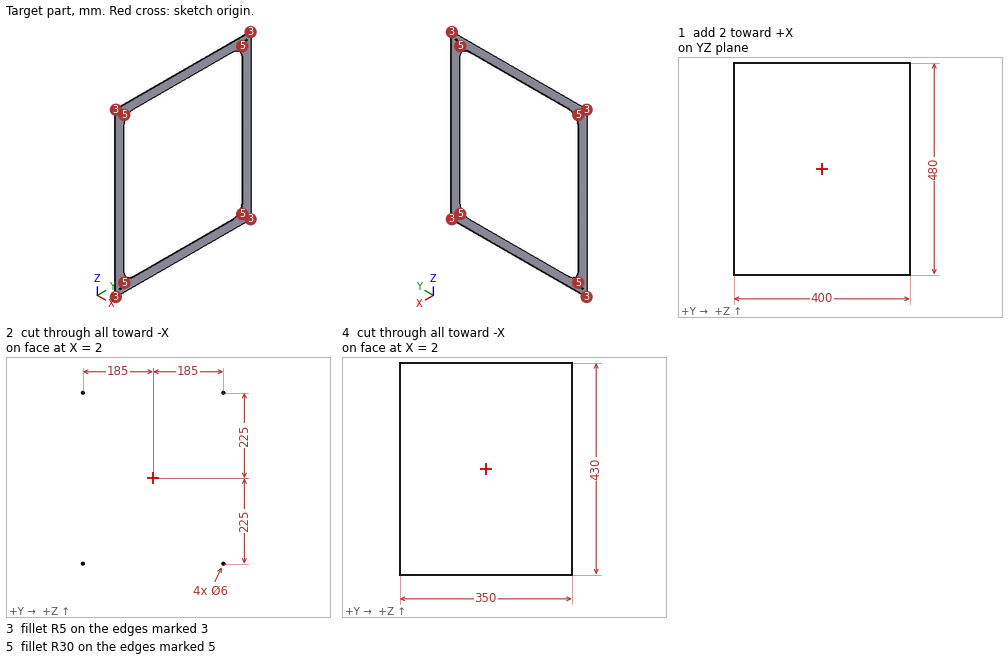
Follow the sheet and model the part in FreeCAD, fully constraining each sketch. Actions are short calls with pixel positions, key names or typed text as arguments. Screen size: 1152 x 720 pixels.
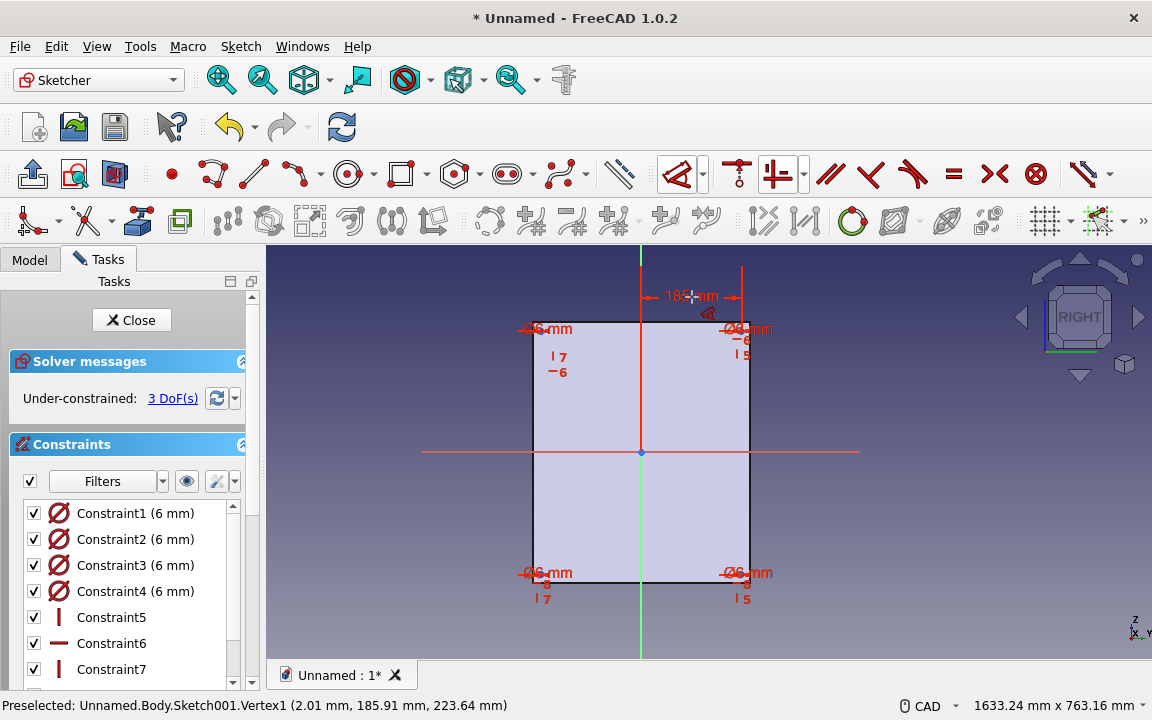
click(742, 331)
click(776, 392)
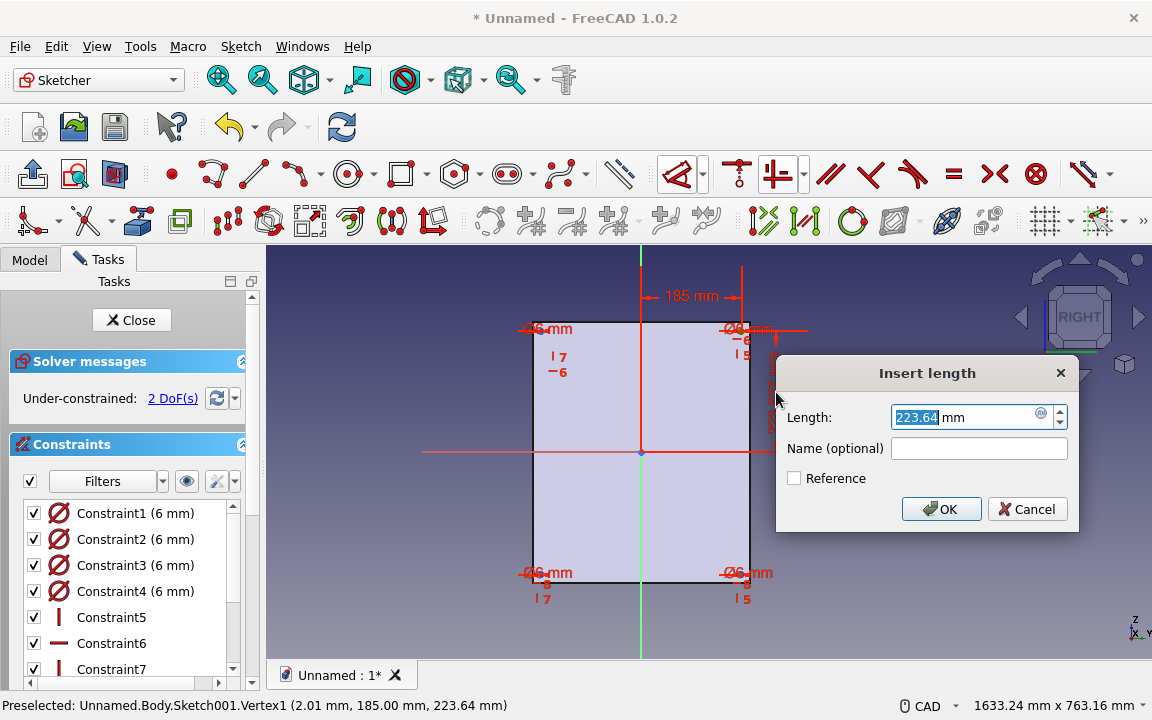
text(225)
key(Return)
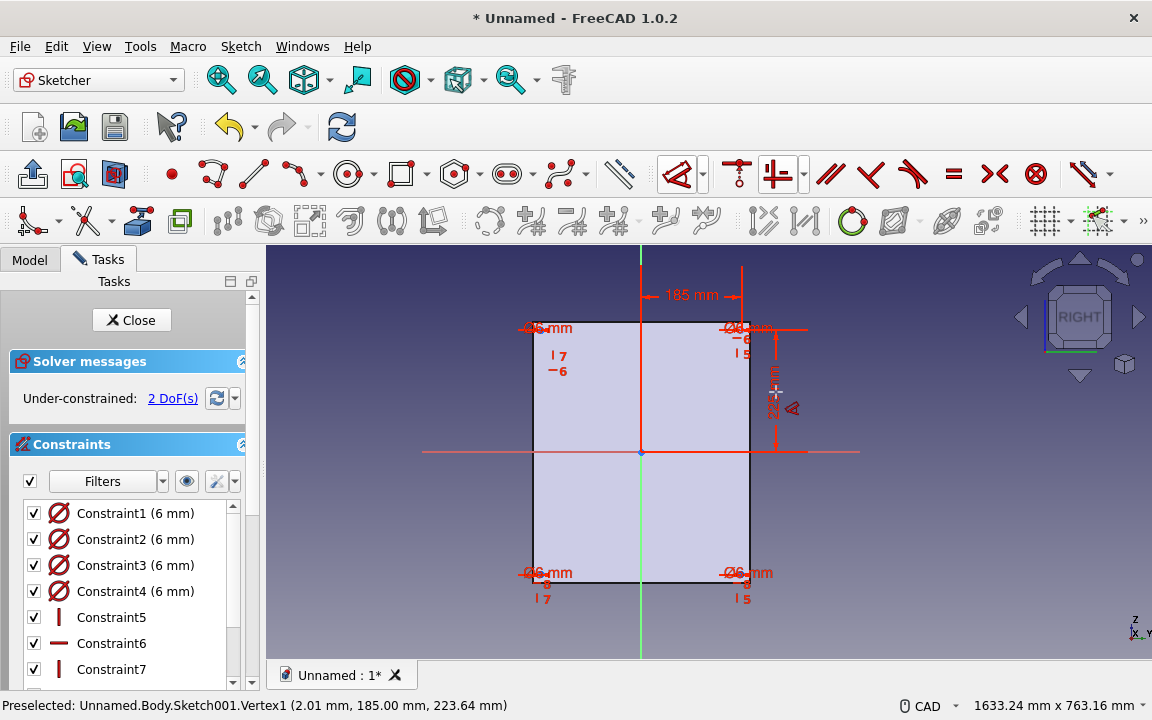
click(742, 575)
click(776, 514)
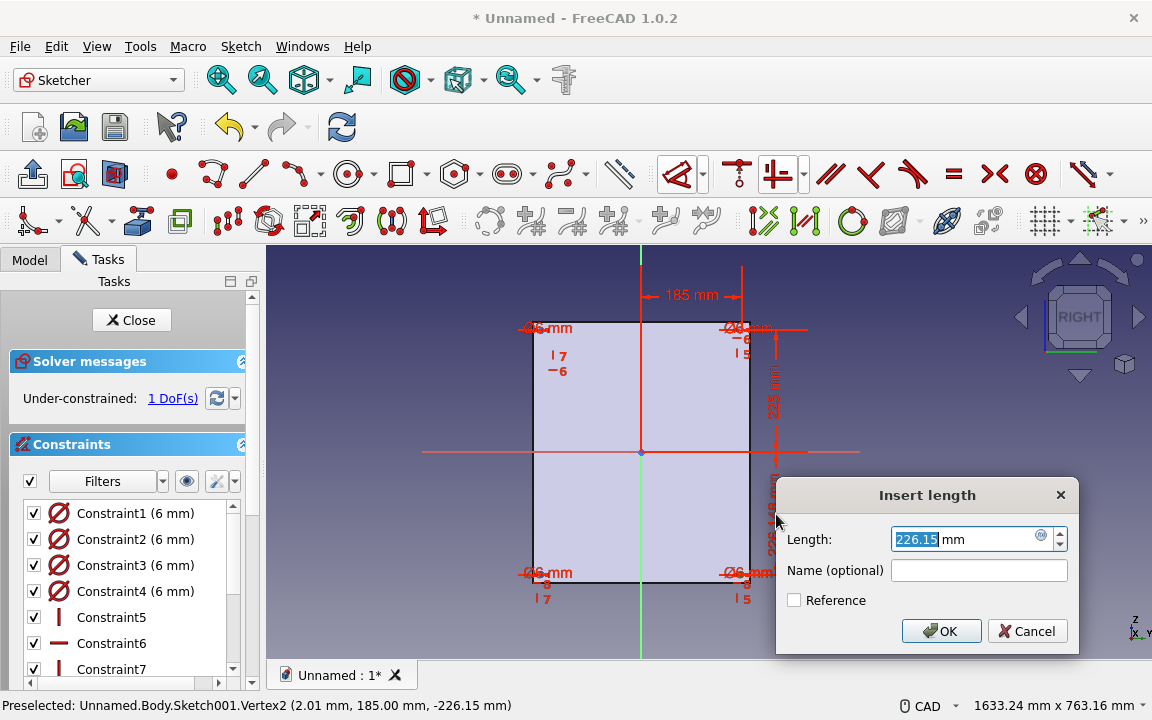
text(225)
key(Return)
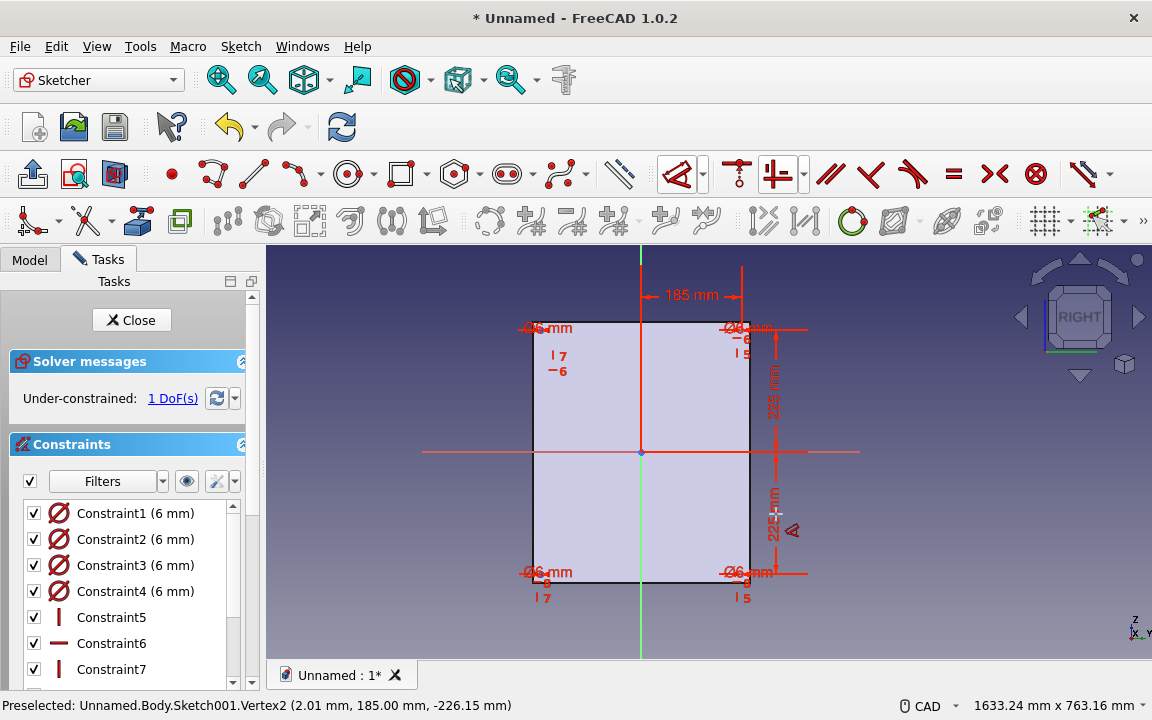
click(541, 330)
click(591, 296)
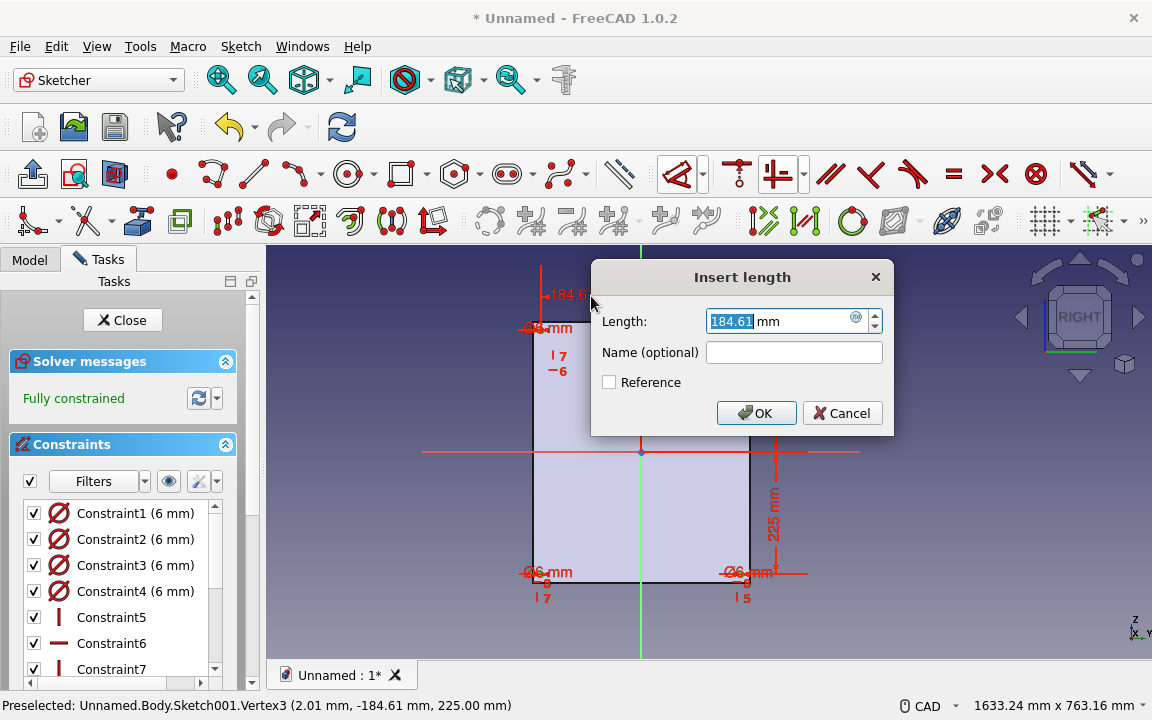
text(185)
key(Return)
key(Escape)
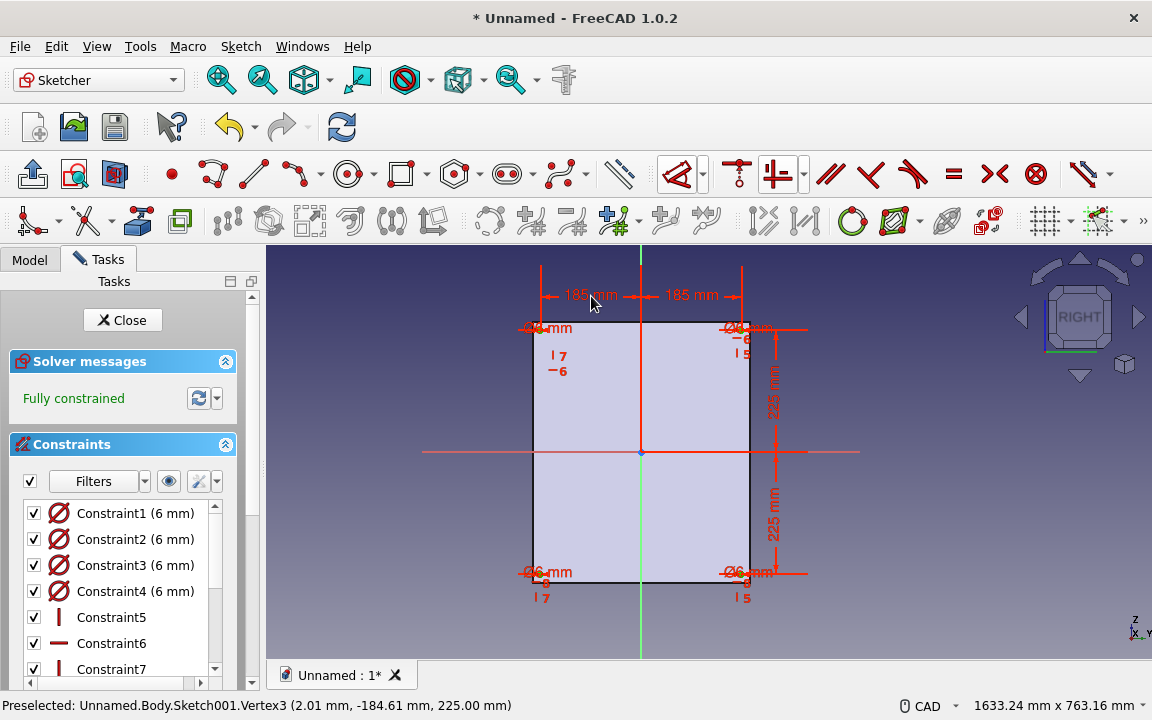
click(123, 320)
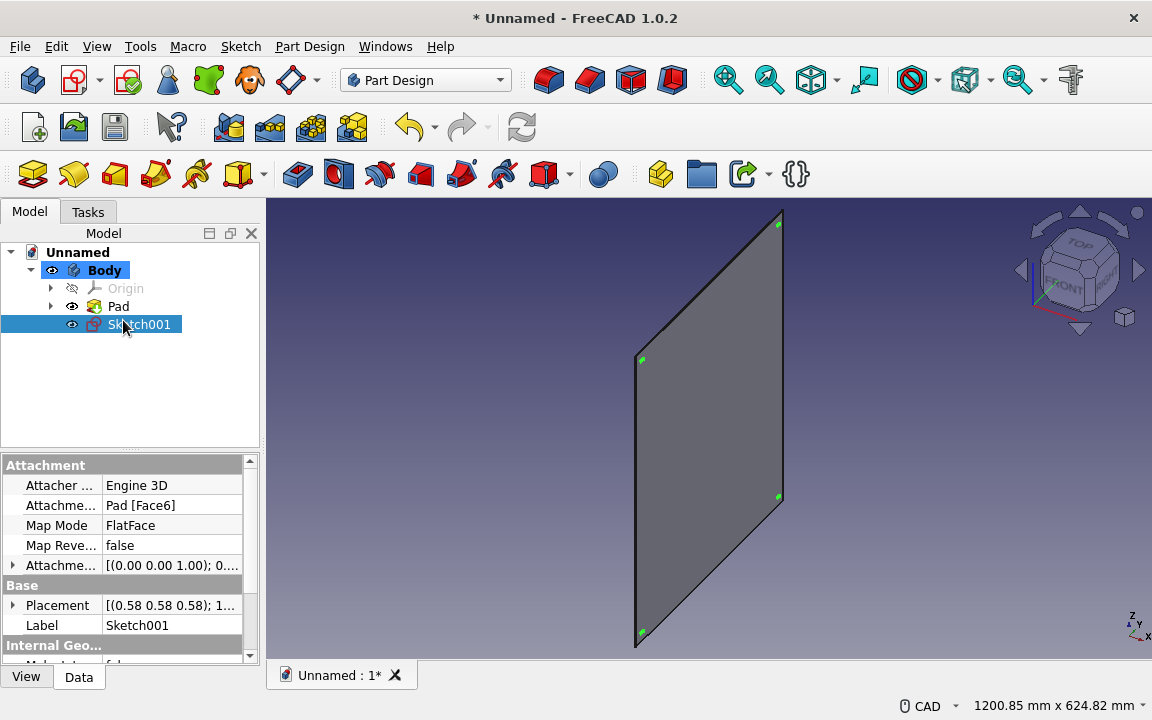
click(298, 174)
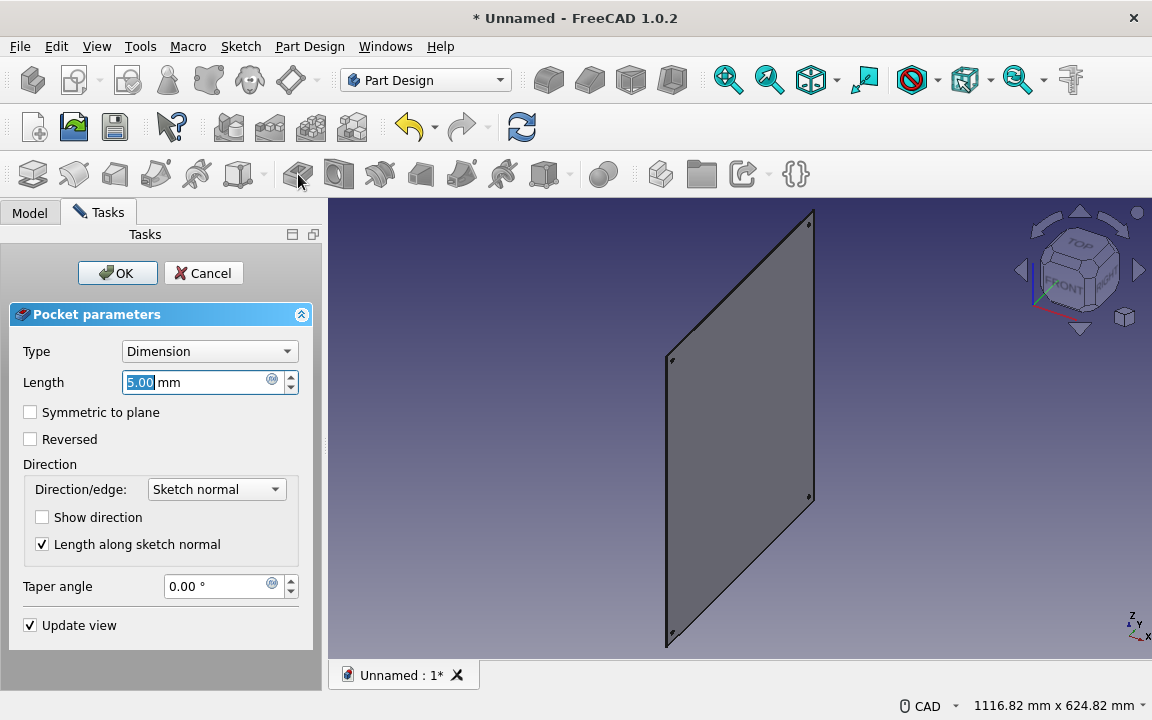
click(210, 352)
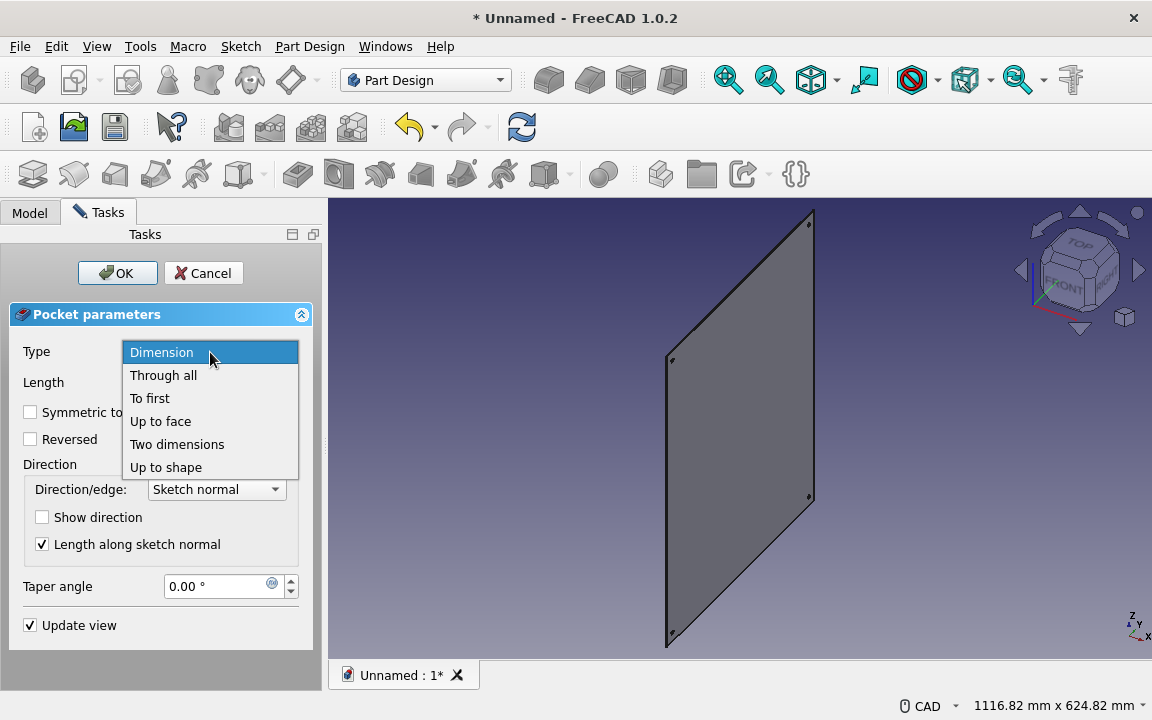
click(208, 376)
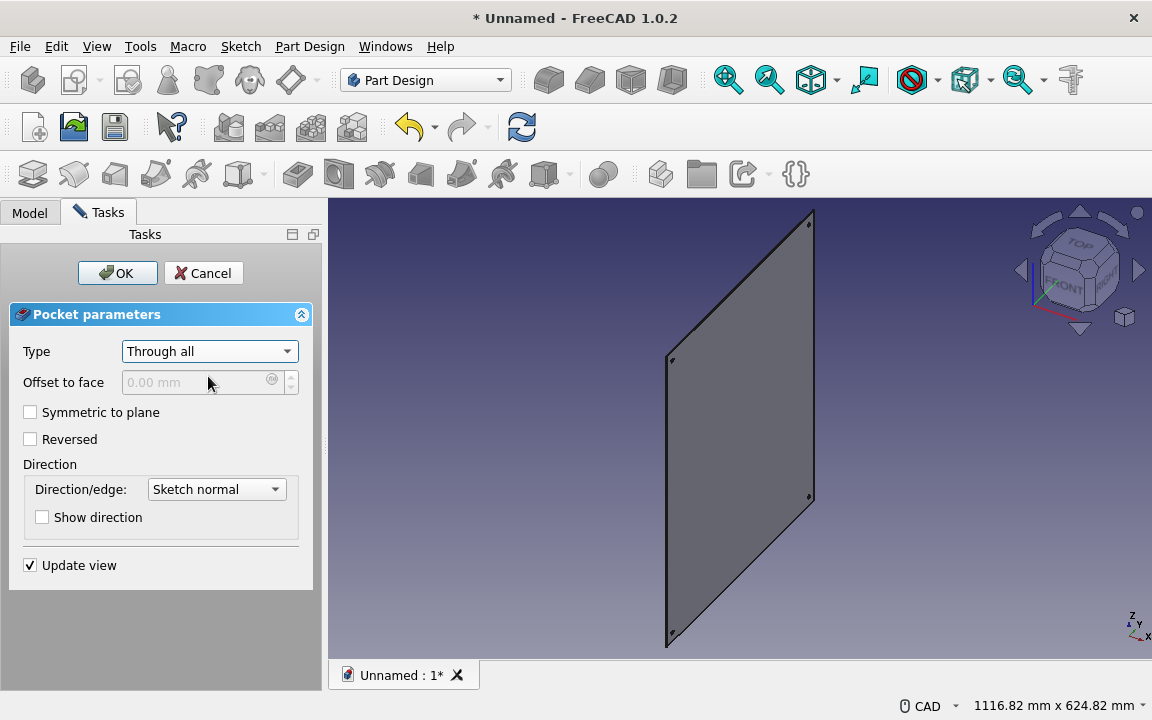
click(118, 273)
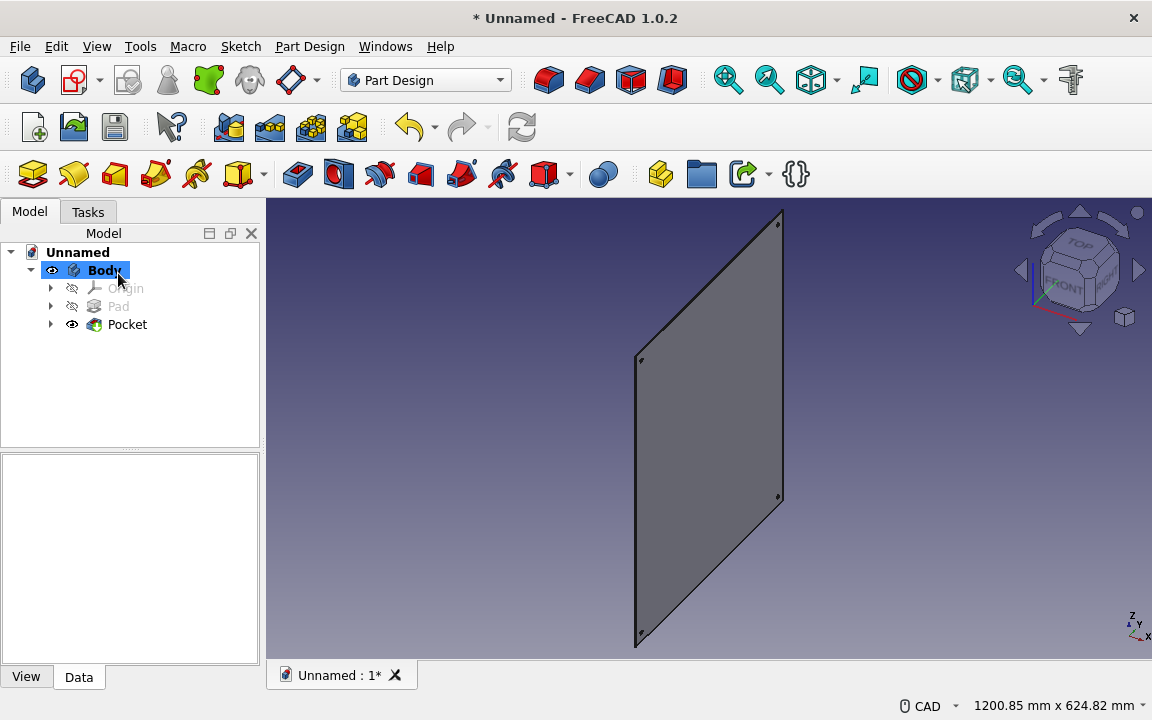
key(0)